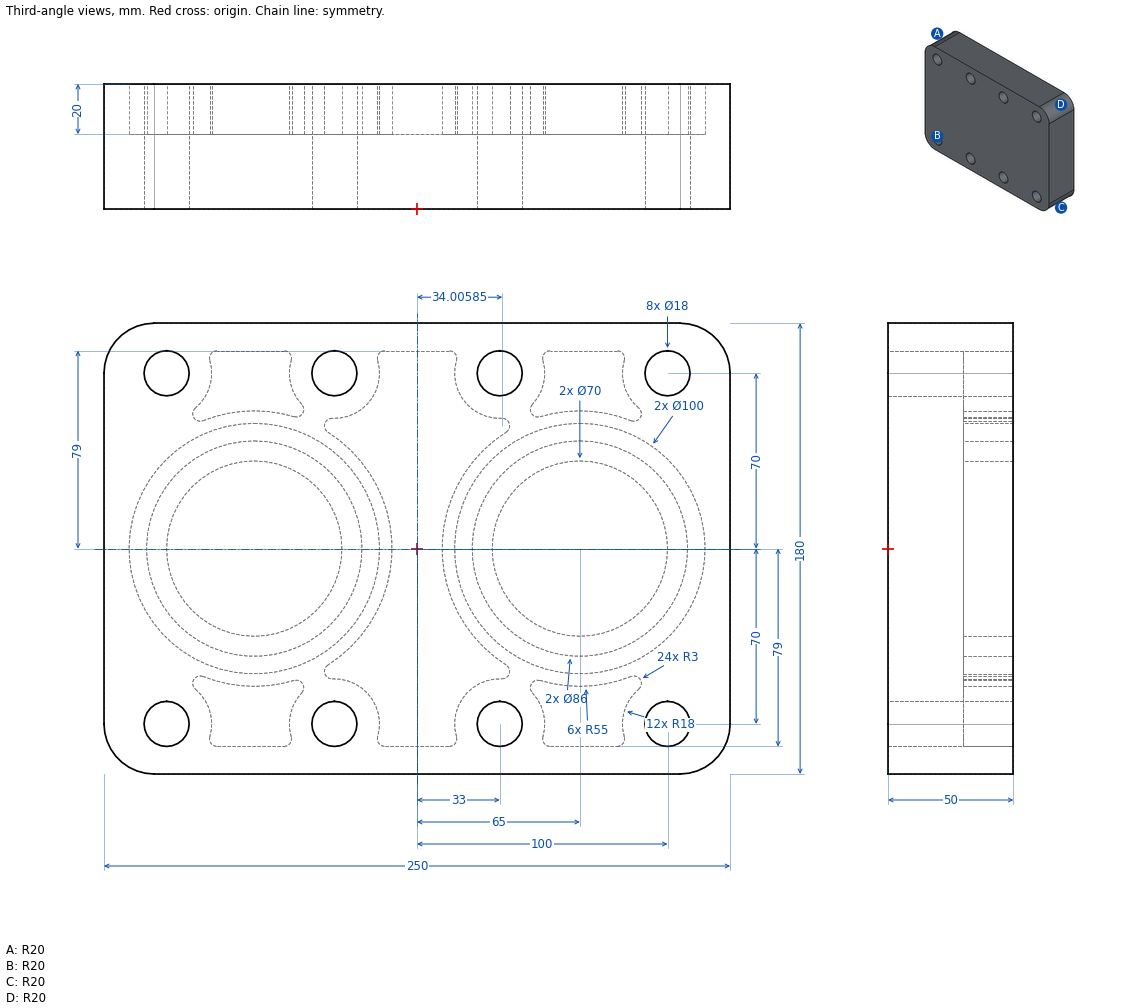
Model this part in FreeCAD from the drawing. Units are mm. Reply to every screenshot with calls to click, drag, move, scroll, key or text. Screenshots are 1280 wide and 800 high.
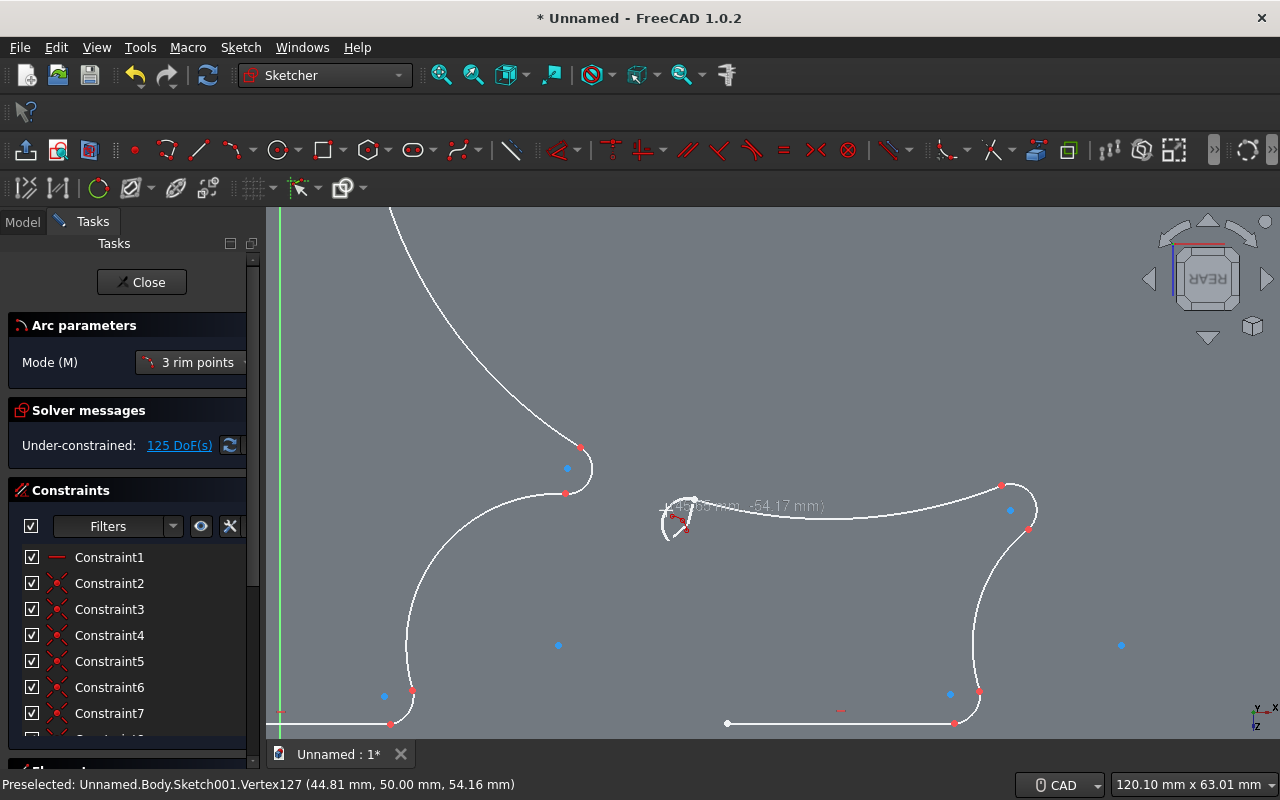
click(666, 509)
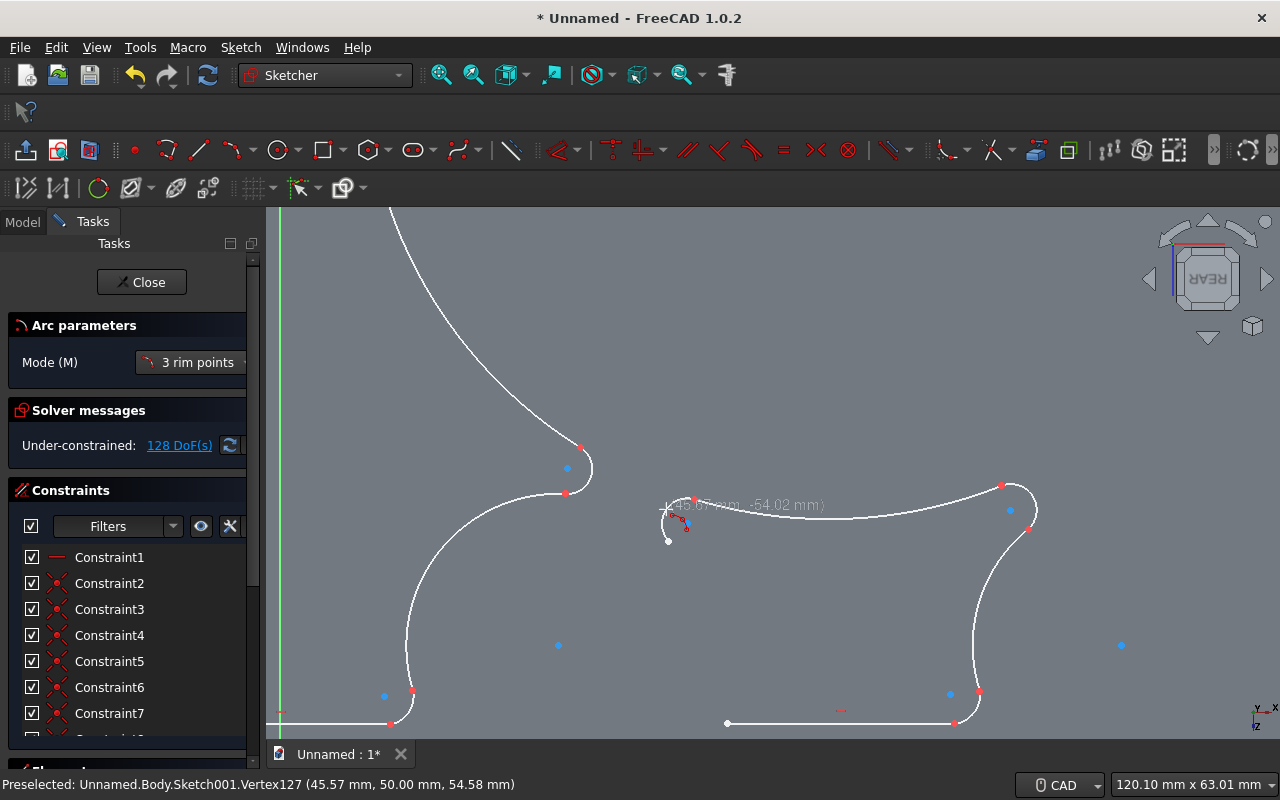
click(669, 541)
click(705, 688)
click(707, 609)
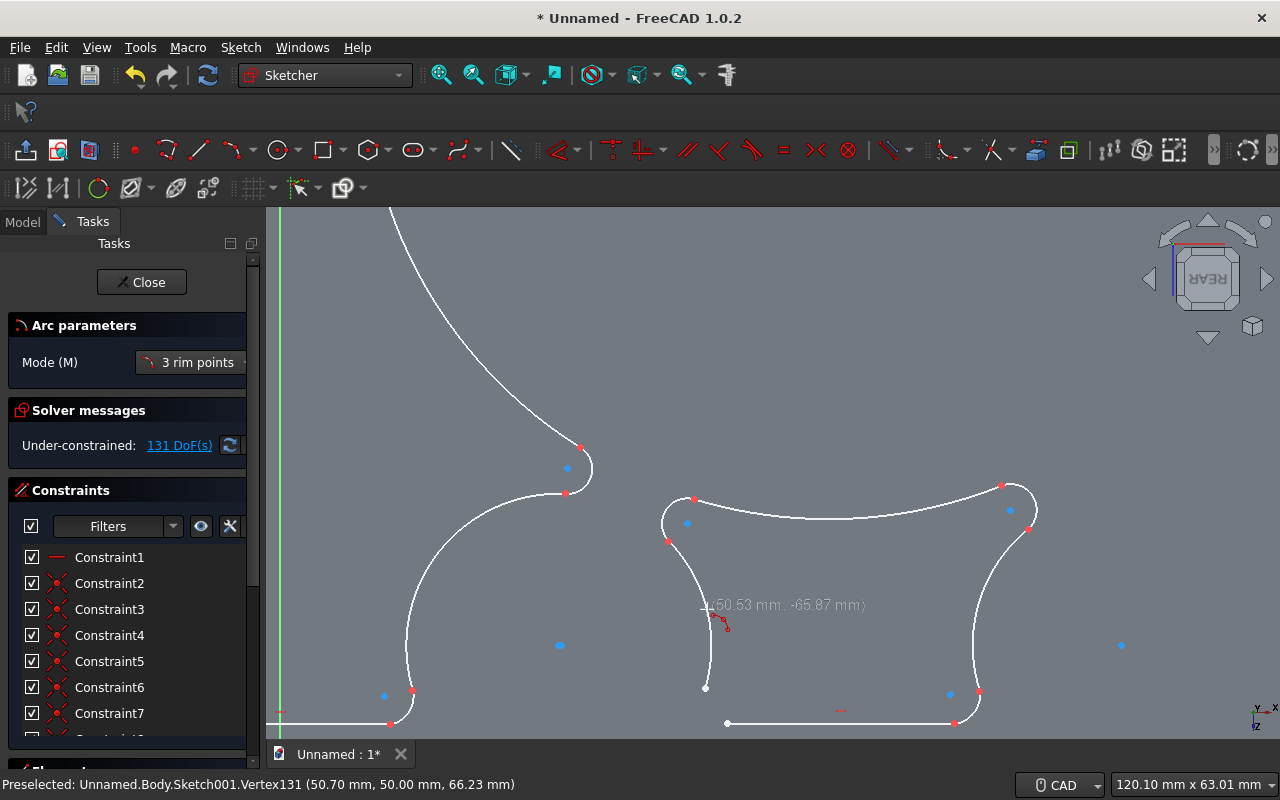
click(705, 689)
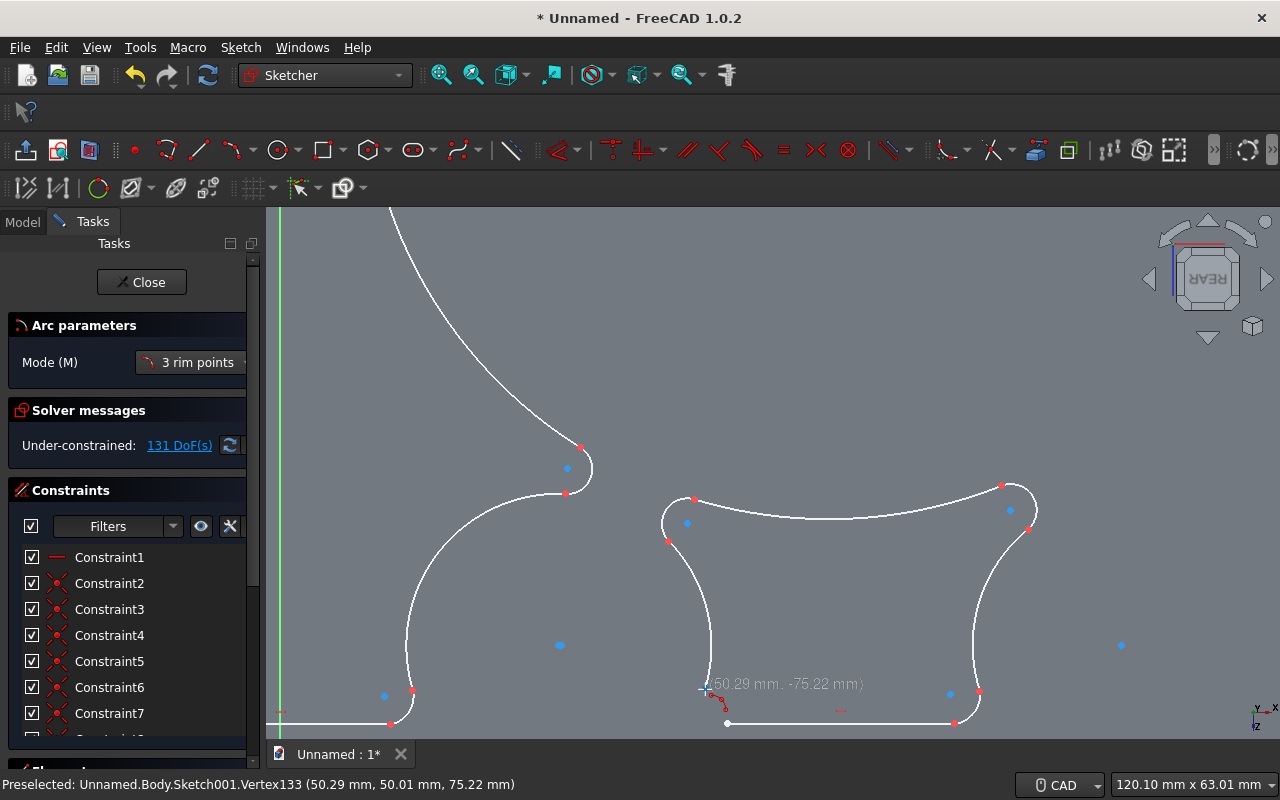
scroll(843, 610, down, 7)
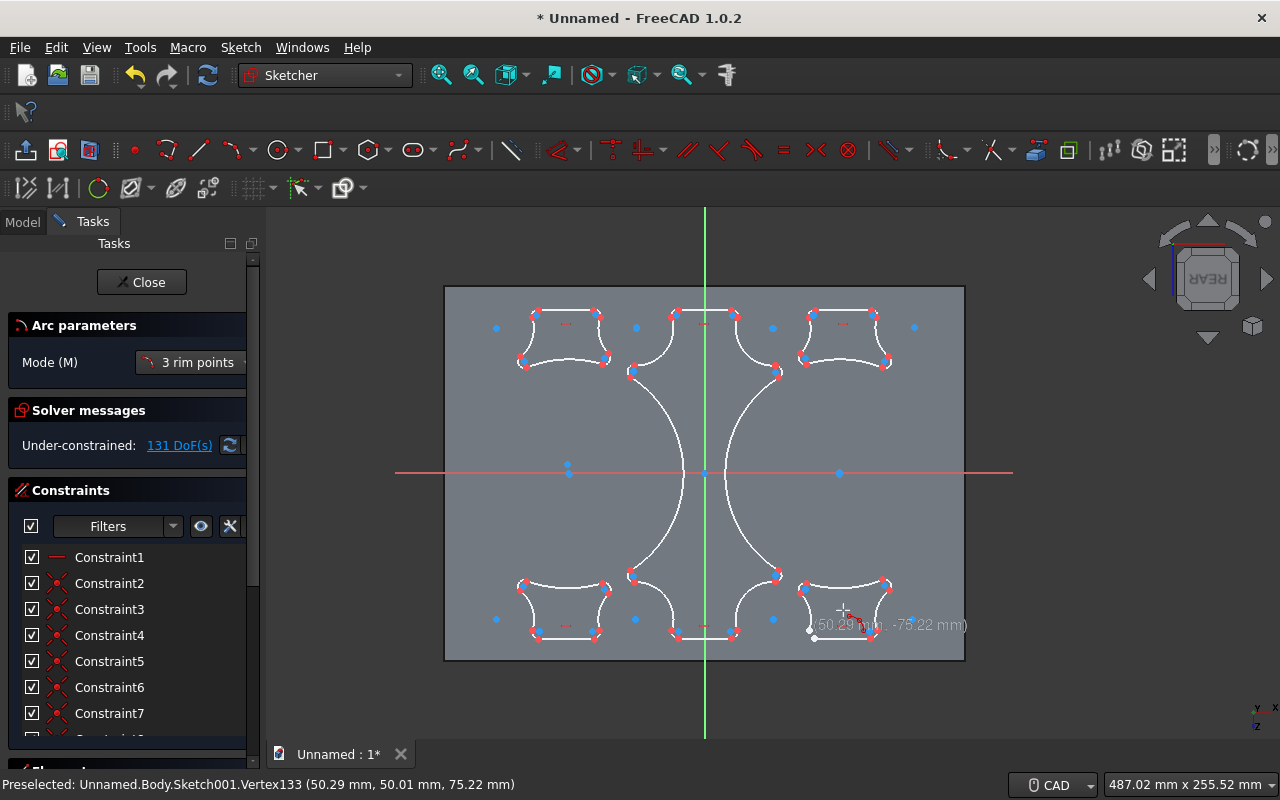
scroll(815, 638, up, 3)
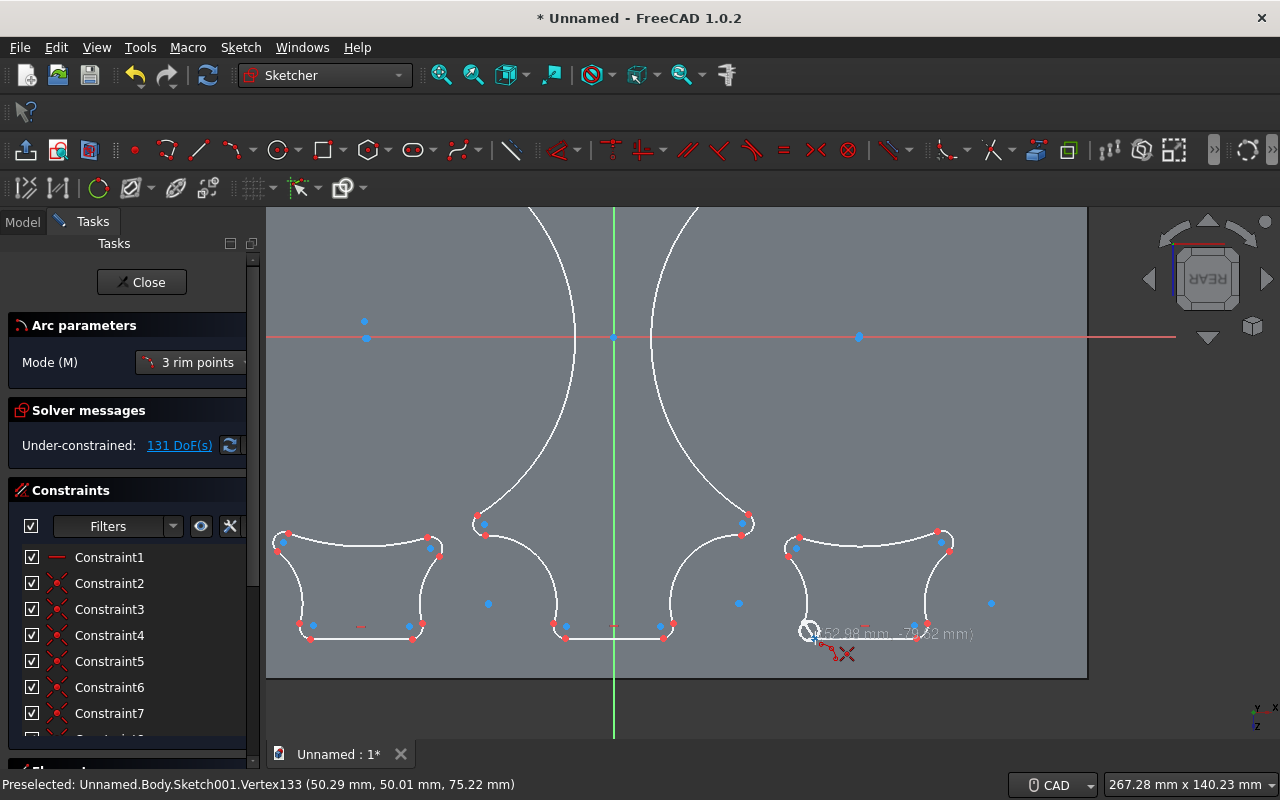
click(814, 639)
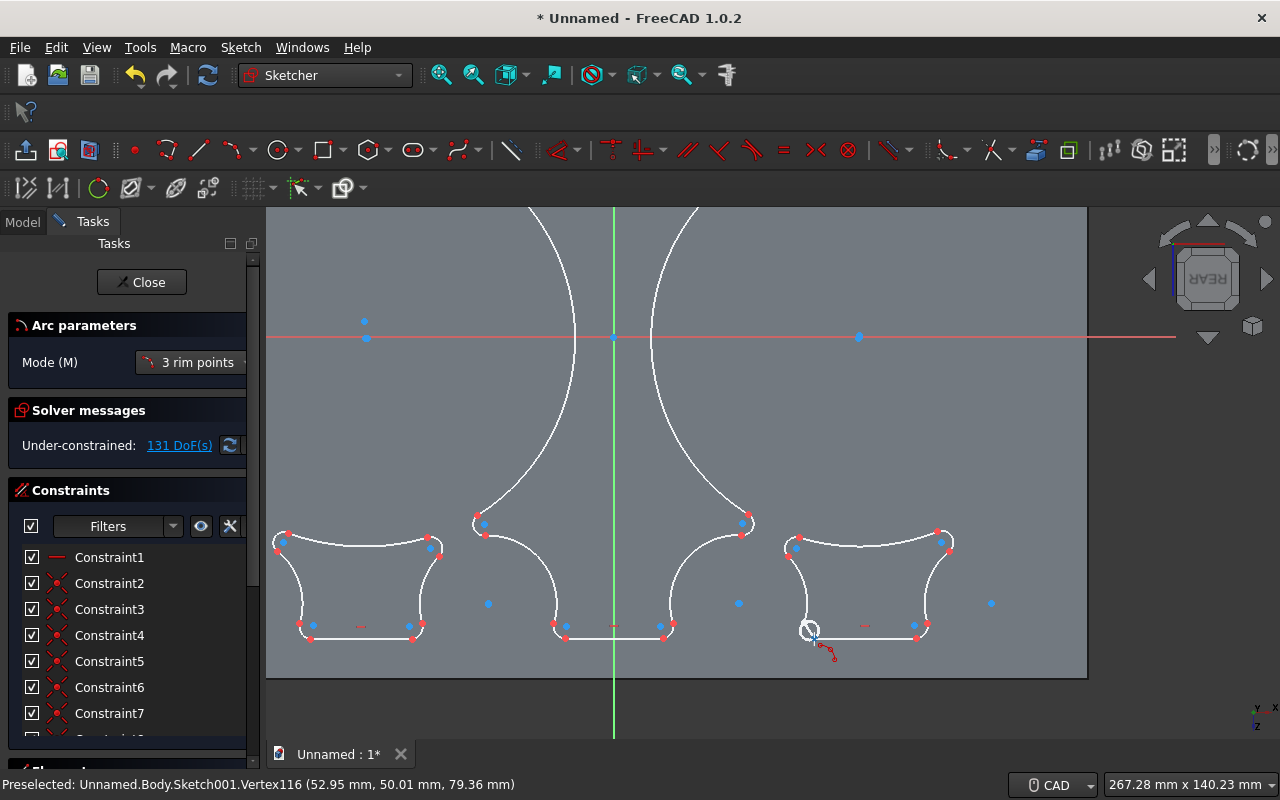
scroll(806, 633, up, 7)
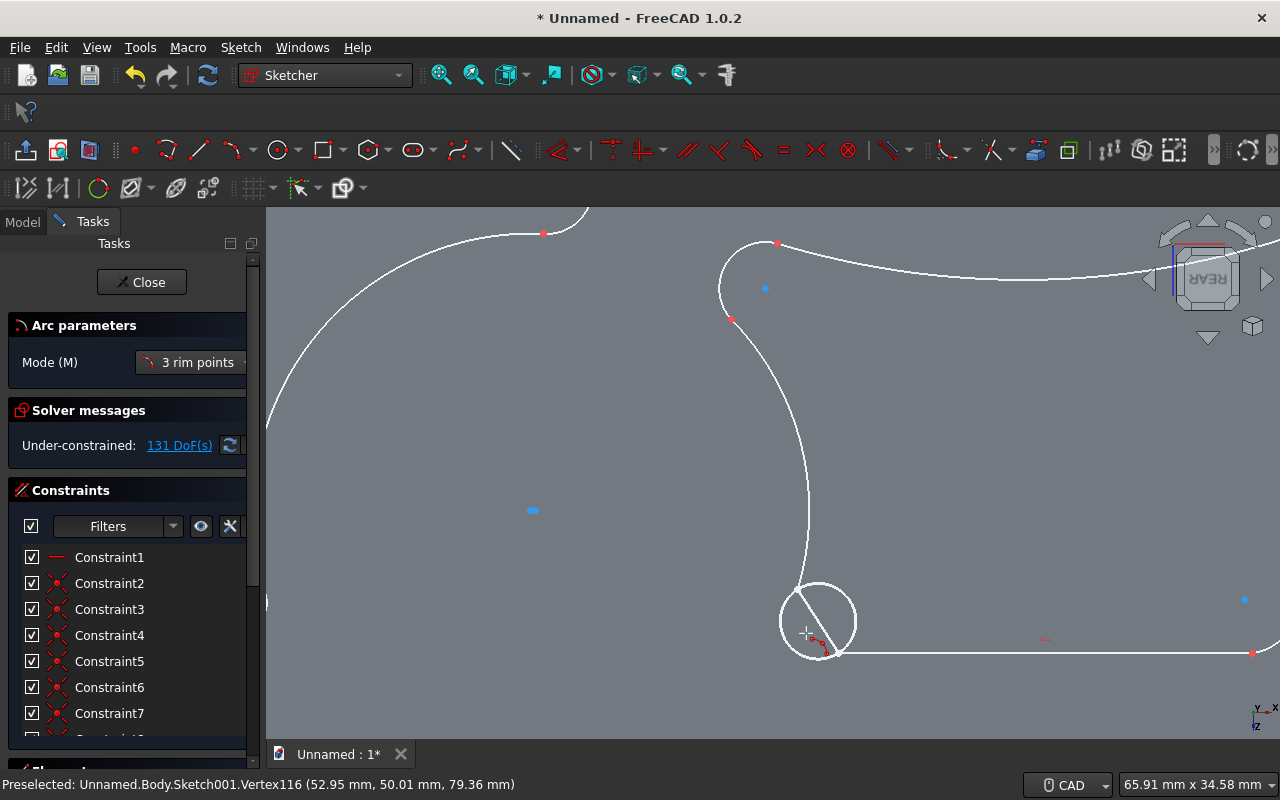
click(804, 629)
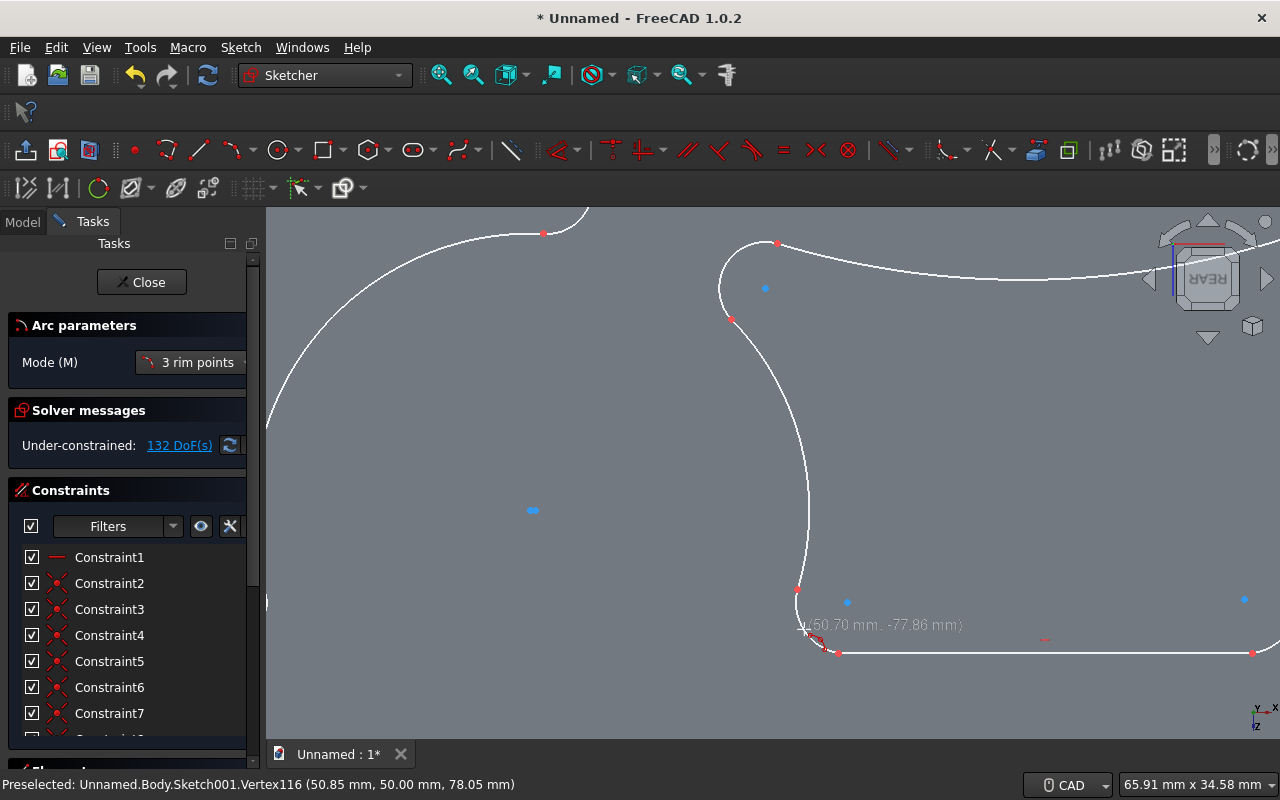
click(278, 150)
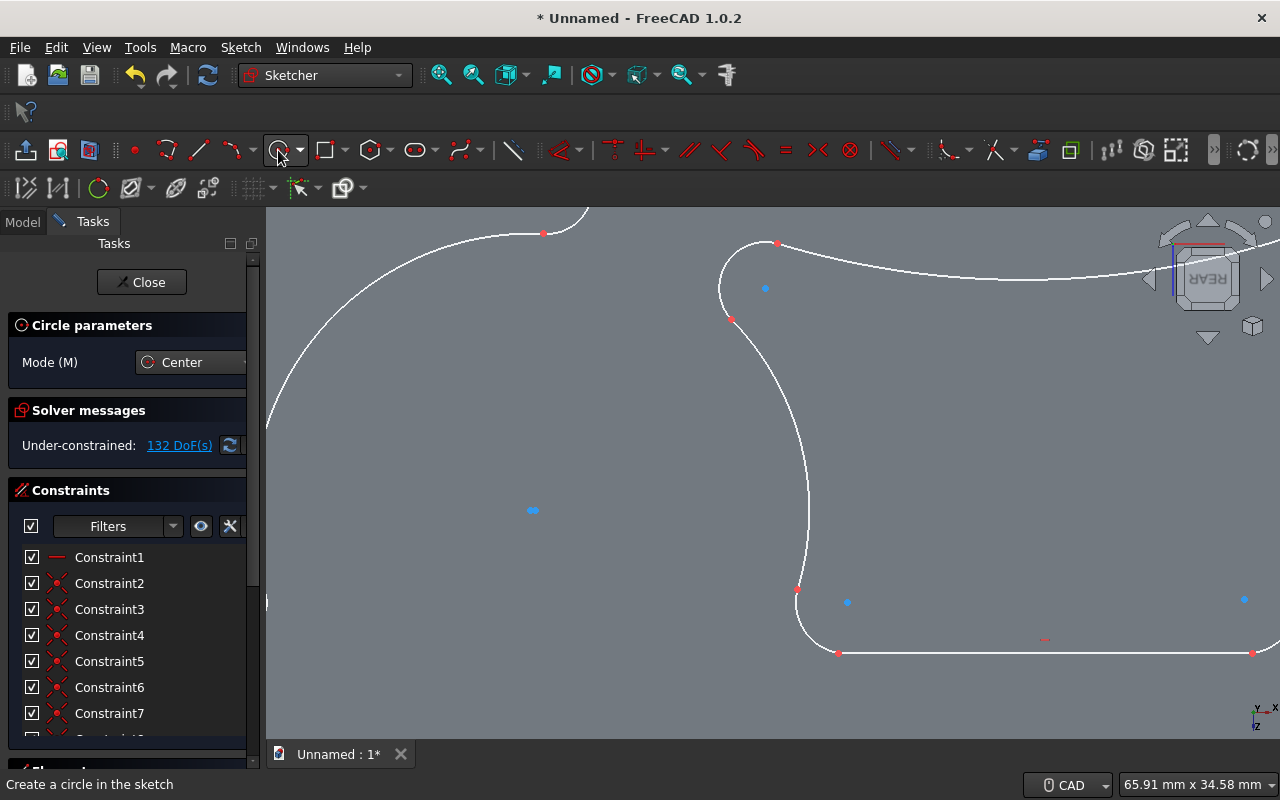
scroll(811, 636, down, 10)